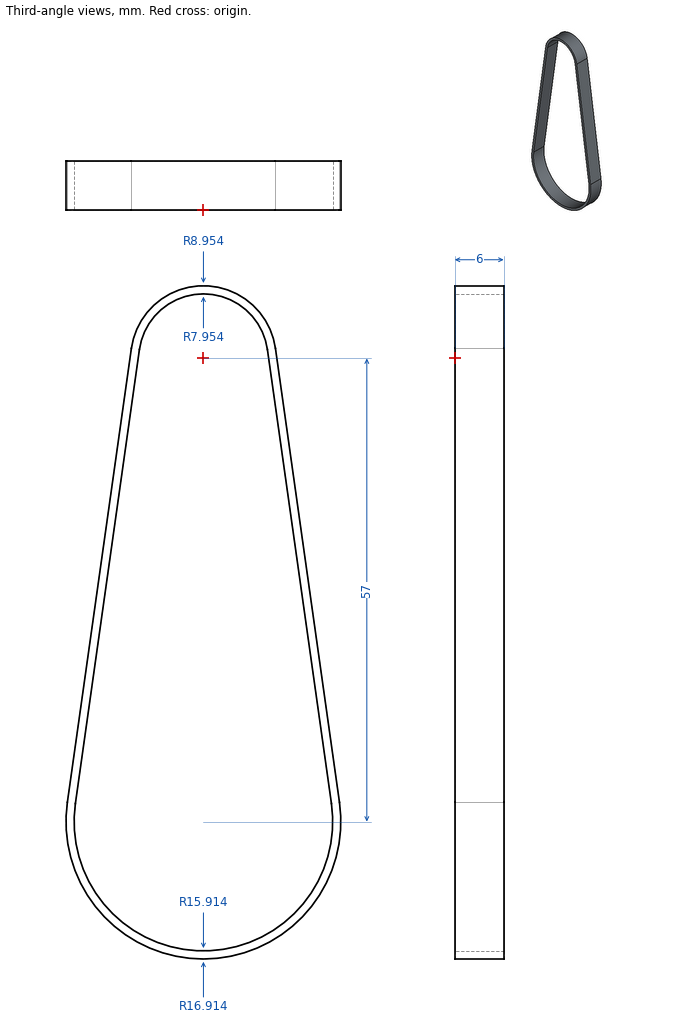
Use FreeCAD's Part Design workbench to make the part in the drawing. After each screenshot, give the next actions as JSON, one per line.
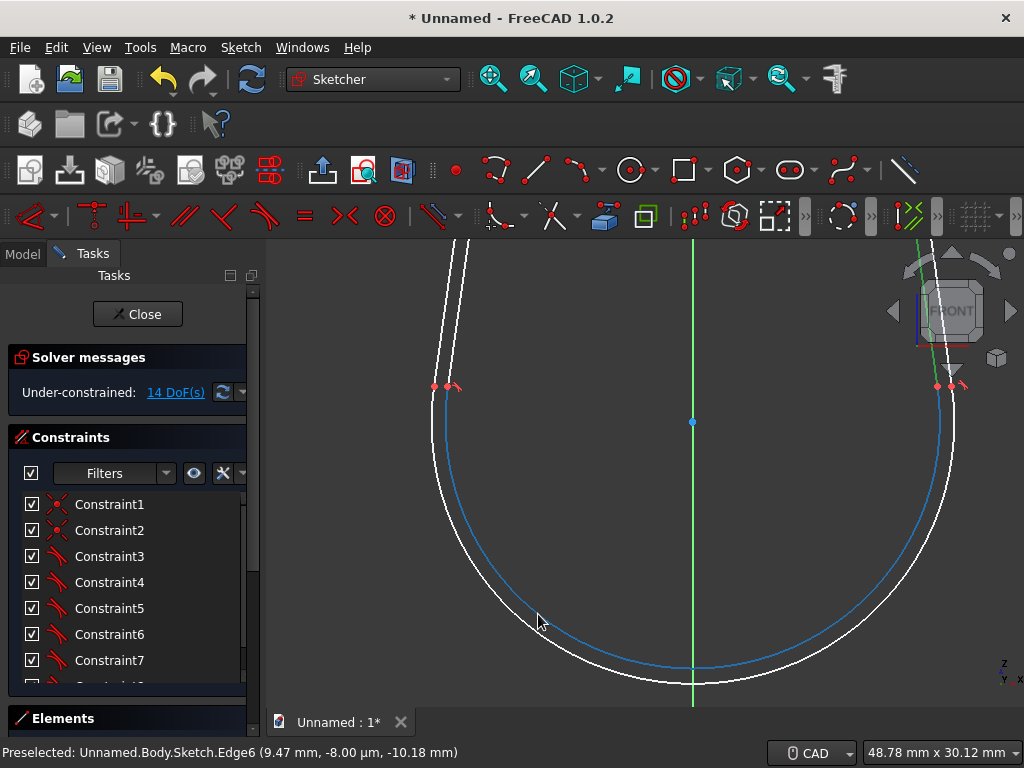
{"action": "left_click", "coordinate": [536, 613]}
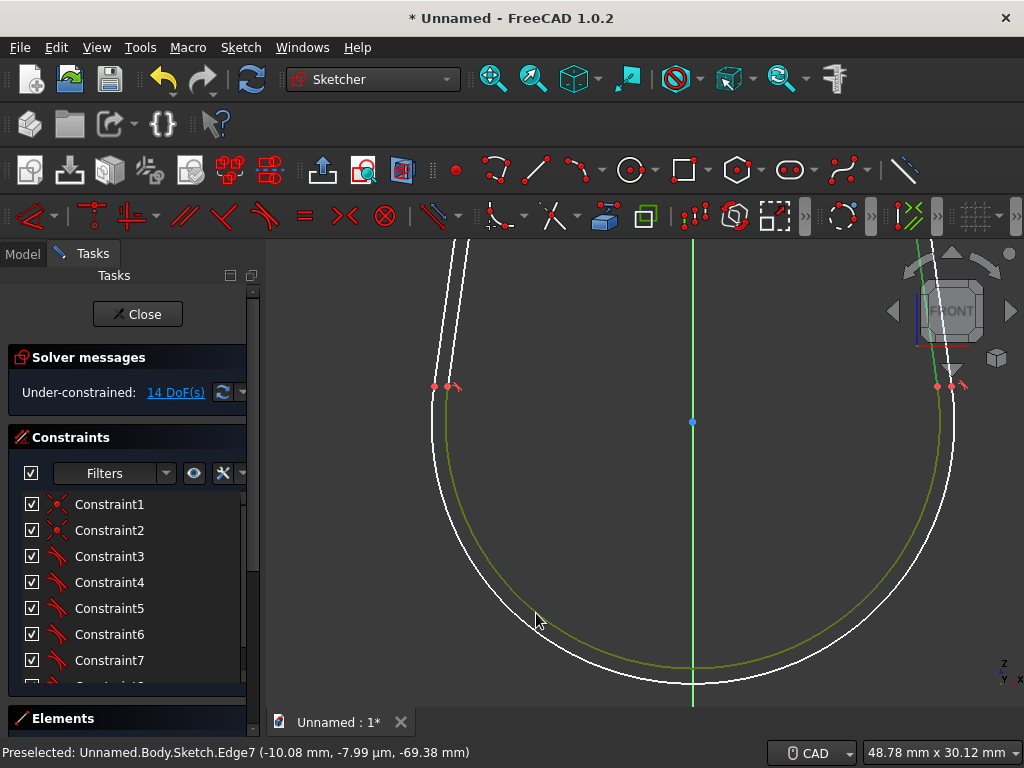
{"action": "left_click", "coordinate": [266, 216]}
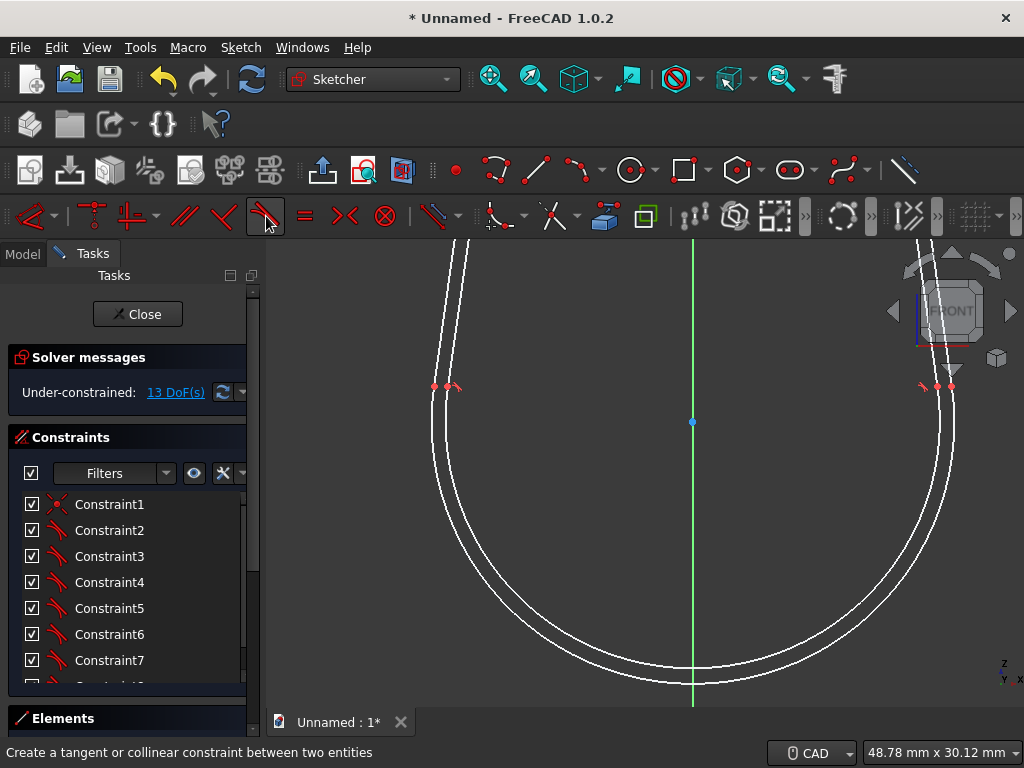
{"action": "scroll", "coordinate": [538, 615], "scroll_direction": "down", "scroll_amount": 7}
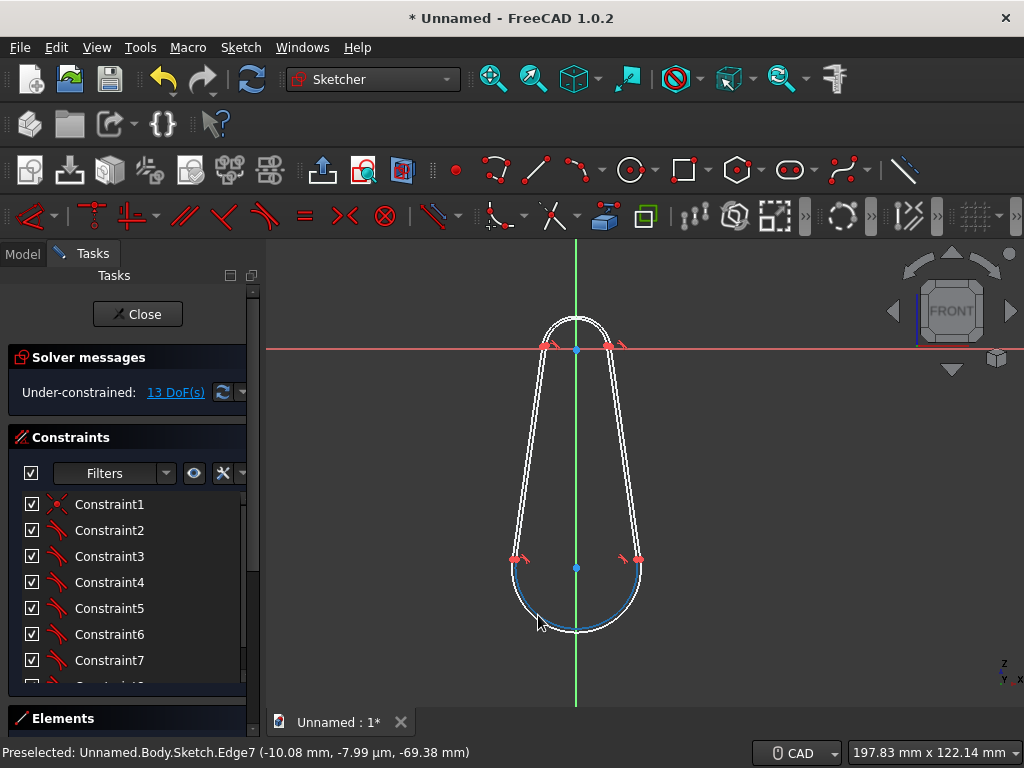
{"action": "scroll", "coordinate": [628, 495], "scroll_direction": "up", "scroll_amount": 7}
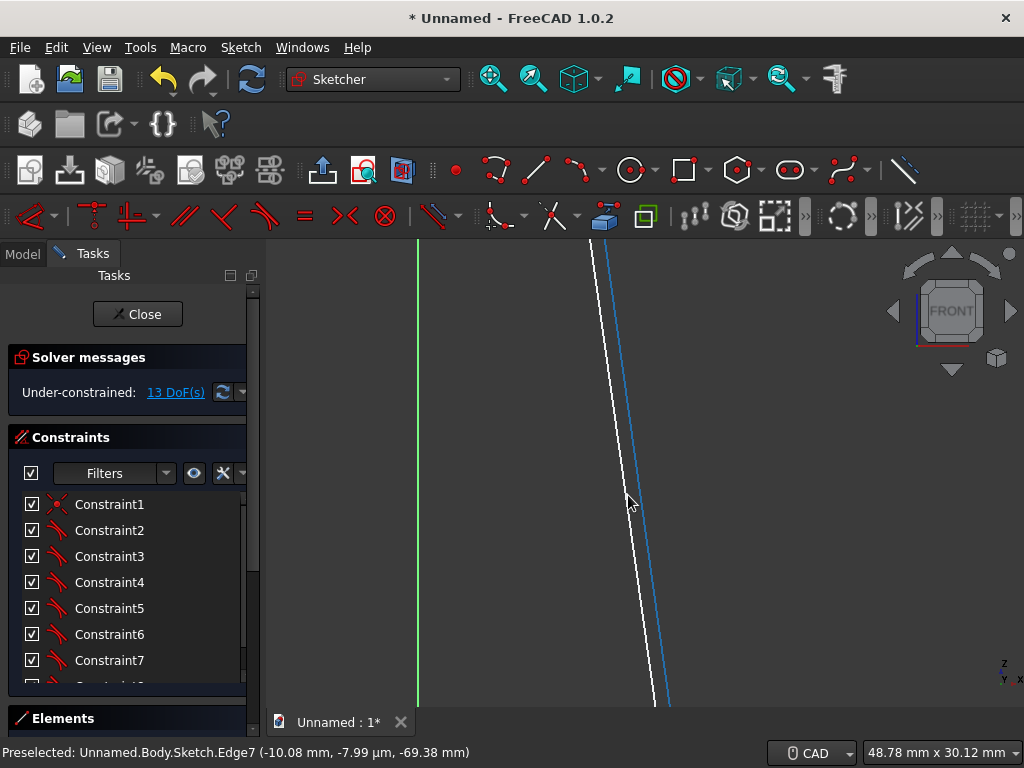
{"action": "left_click", "coordinate": [626, 494]}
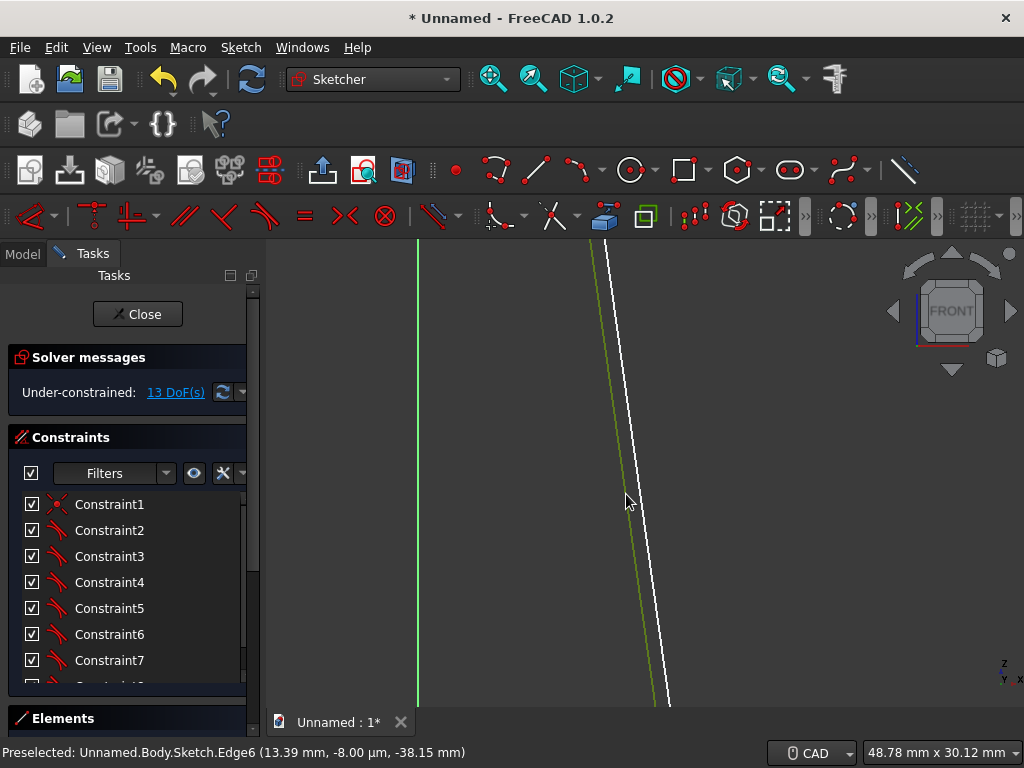
{"action": "scroll", "coordinate": [628, 495], "scroll_direction": "down", "scroll_amount": 7}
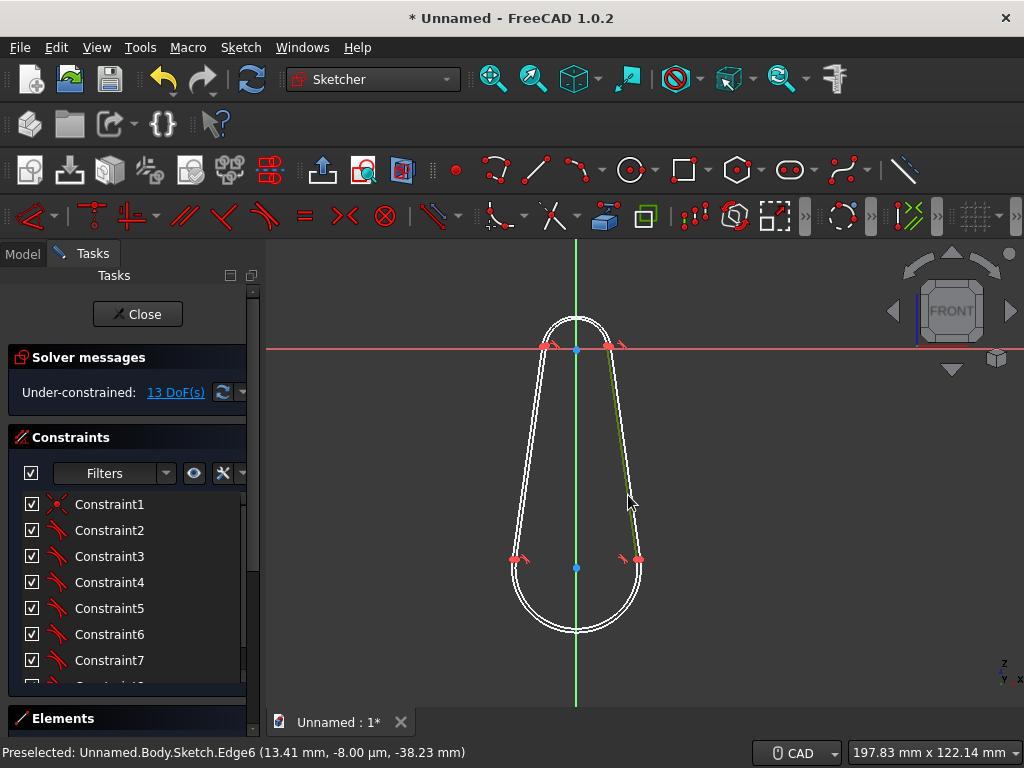
{"action": "scroll", "coordinate": [593, 324], "scroll_direction": "up", "scroll_amount": 9}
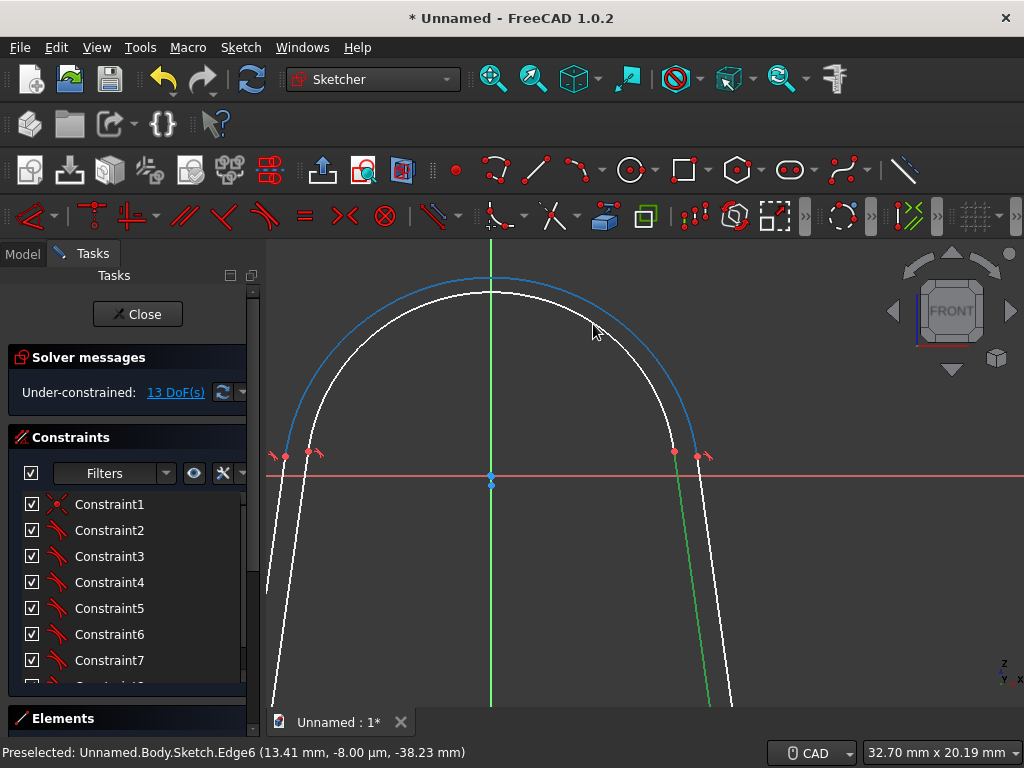
{"action": "left_click", "coordinate": [591, 322]}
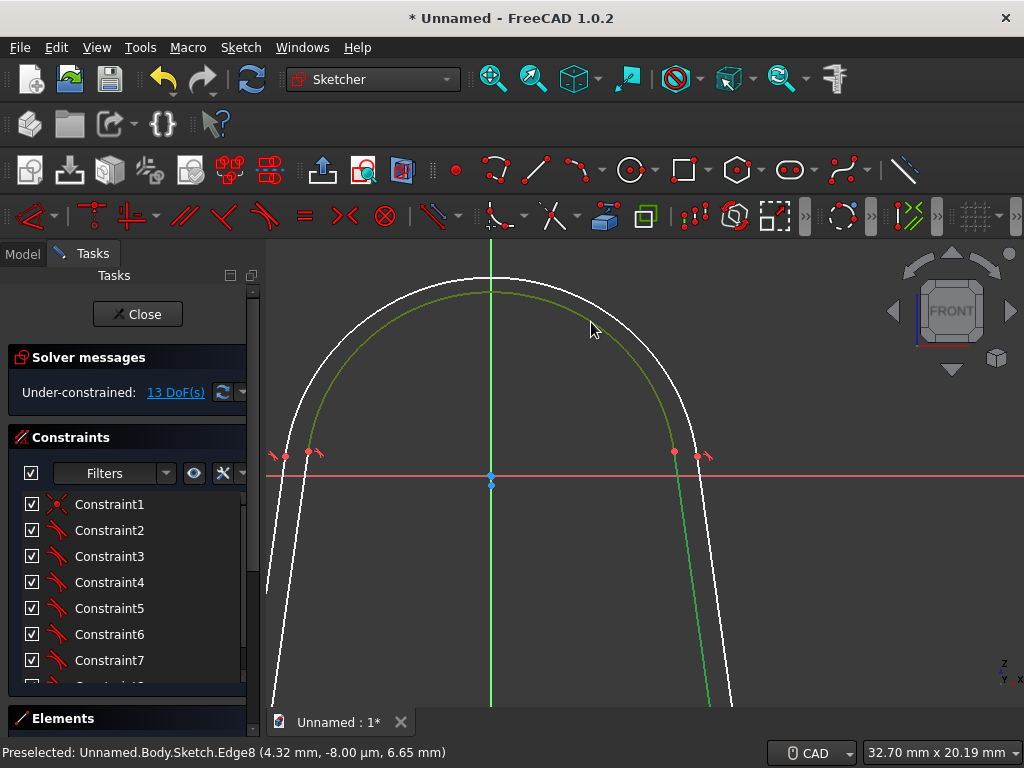
{"action": "left_click", "coordinate": [266, 216]}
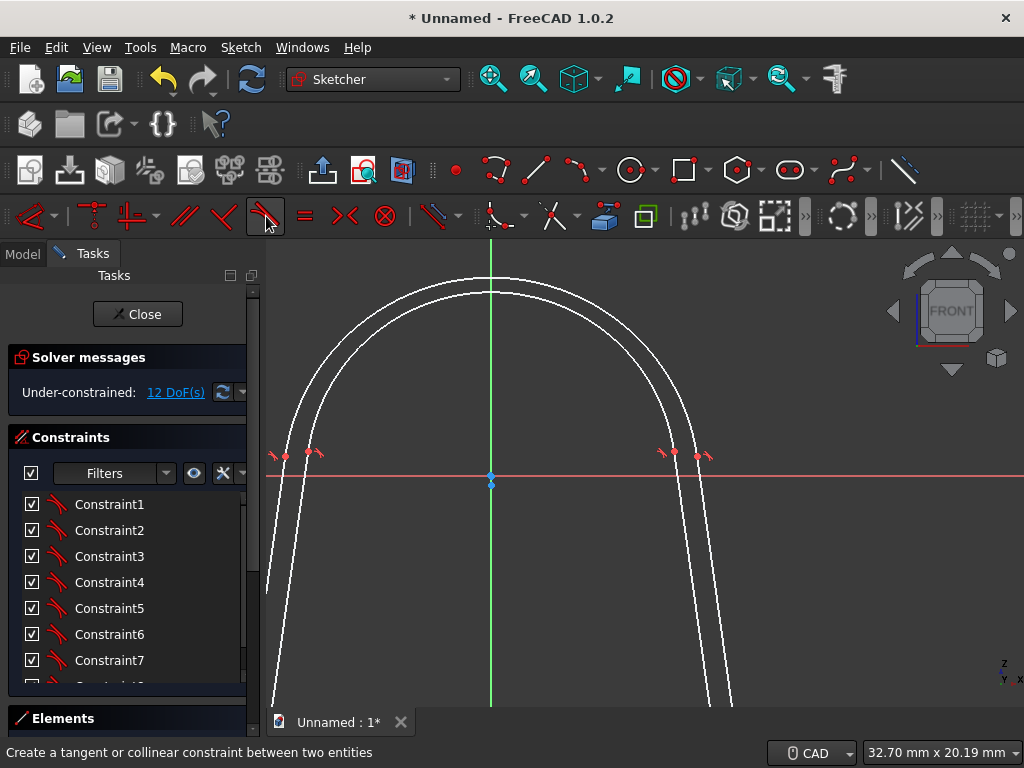
{"action": "scroll", "coordinate": [593, 323], "scroll_direction": "down", "scroll_amount": 9}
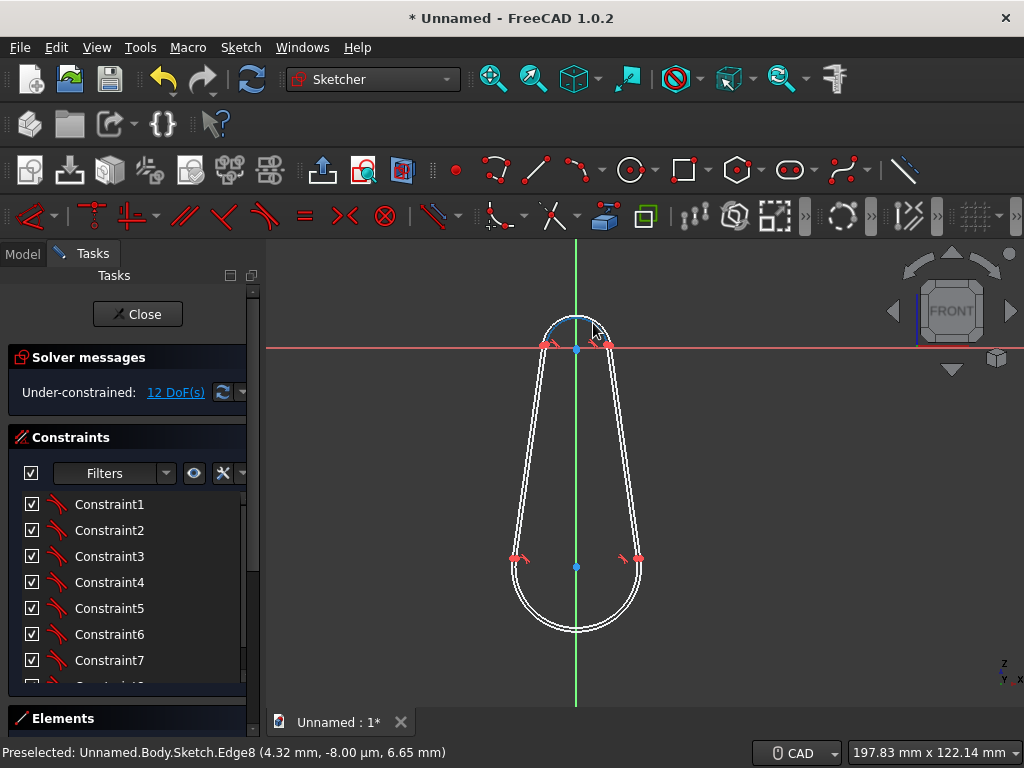
{"action": "scroll", "coordinate": [536, 617], "scroll_direction": "up", "scroll_amount": 7}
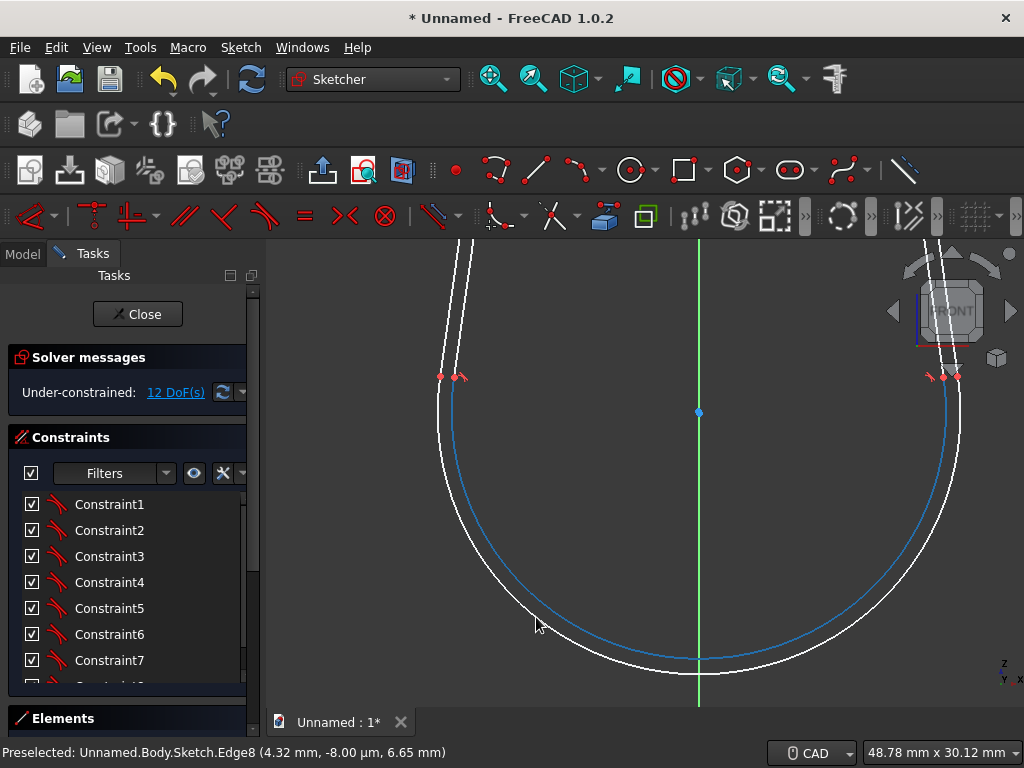
{"action": "left_click", "coordinate": [534, 616]}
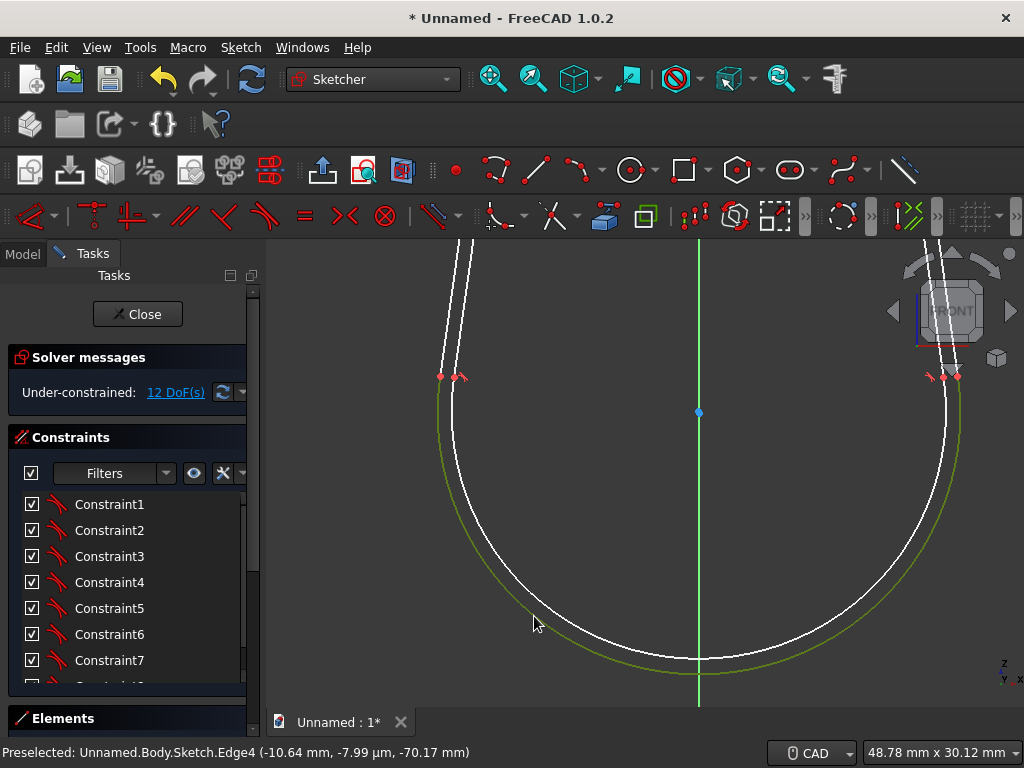
{"action": "left_click", "coordinate": [542, 603]}